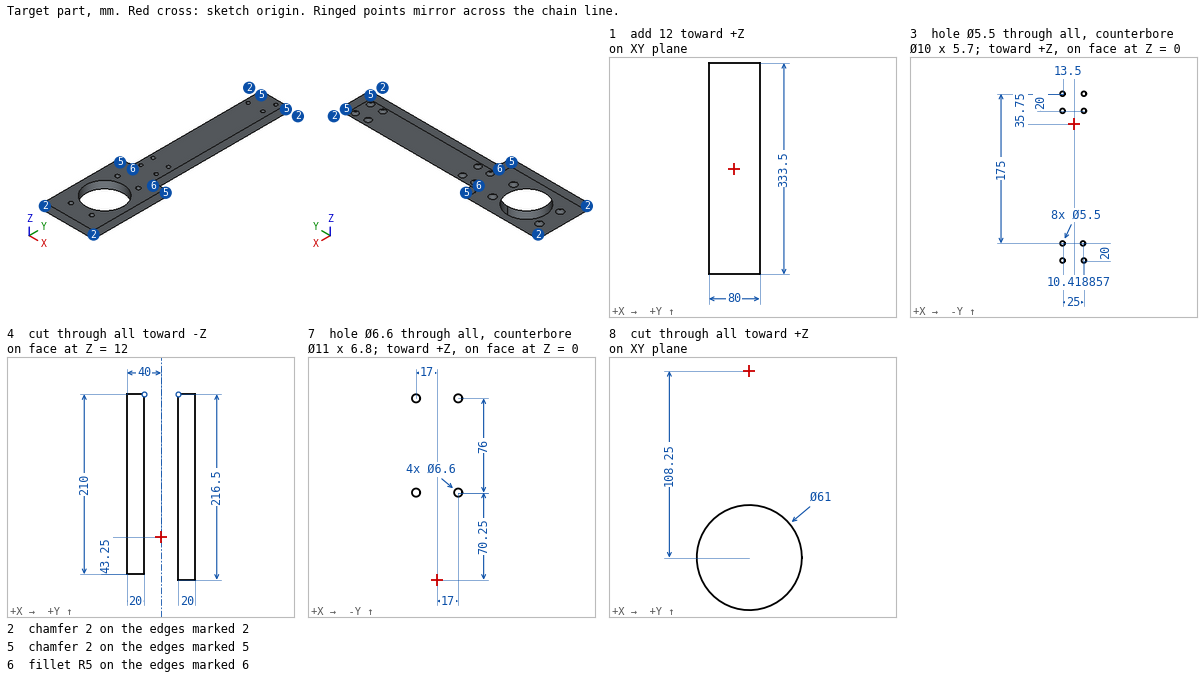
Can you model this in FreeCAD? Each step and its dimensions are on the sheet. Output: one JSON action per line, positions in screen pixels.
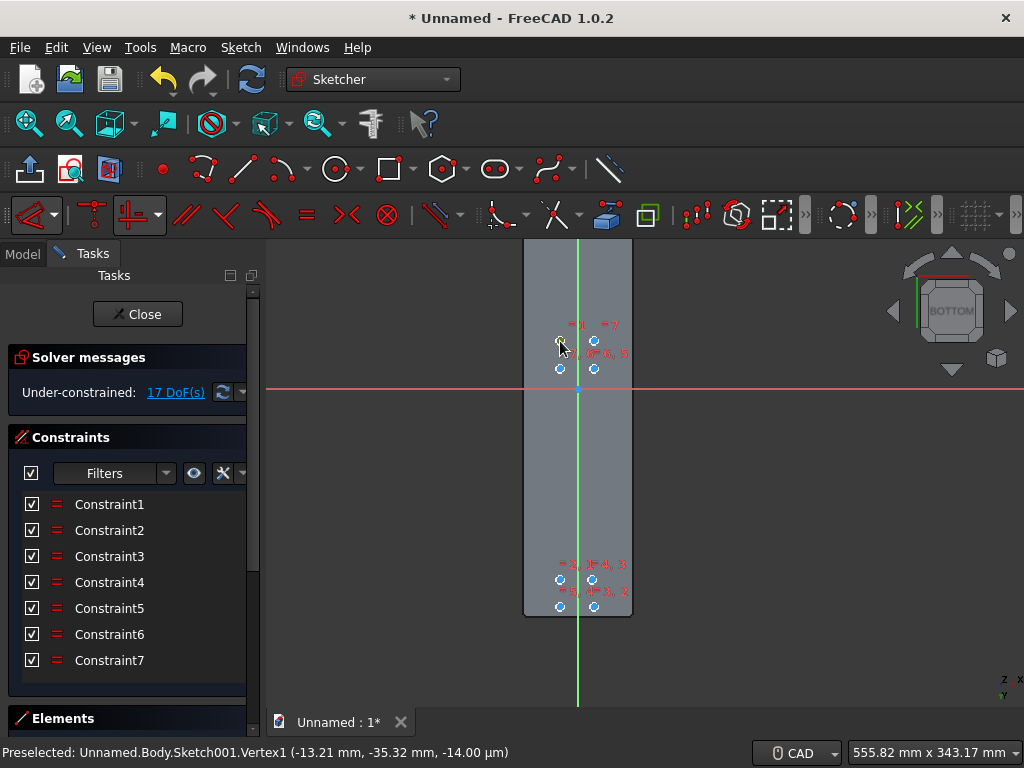
{"action": "left_click", "coordinate": [560, 580]}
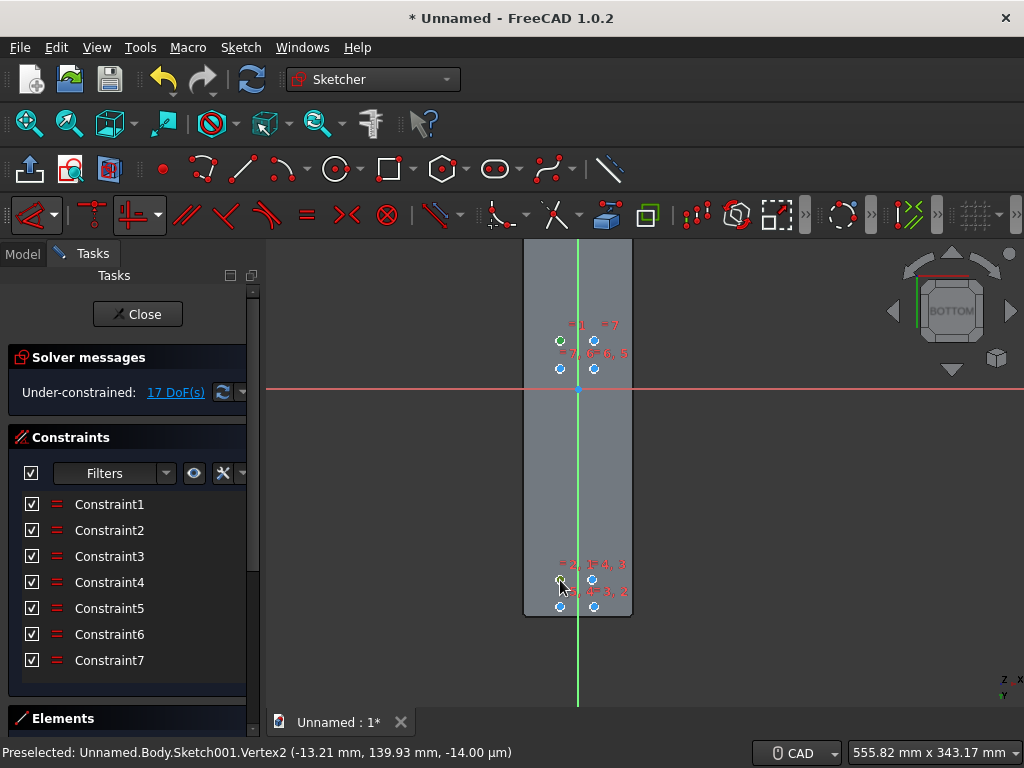
{"action": "key", "text": "v"}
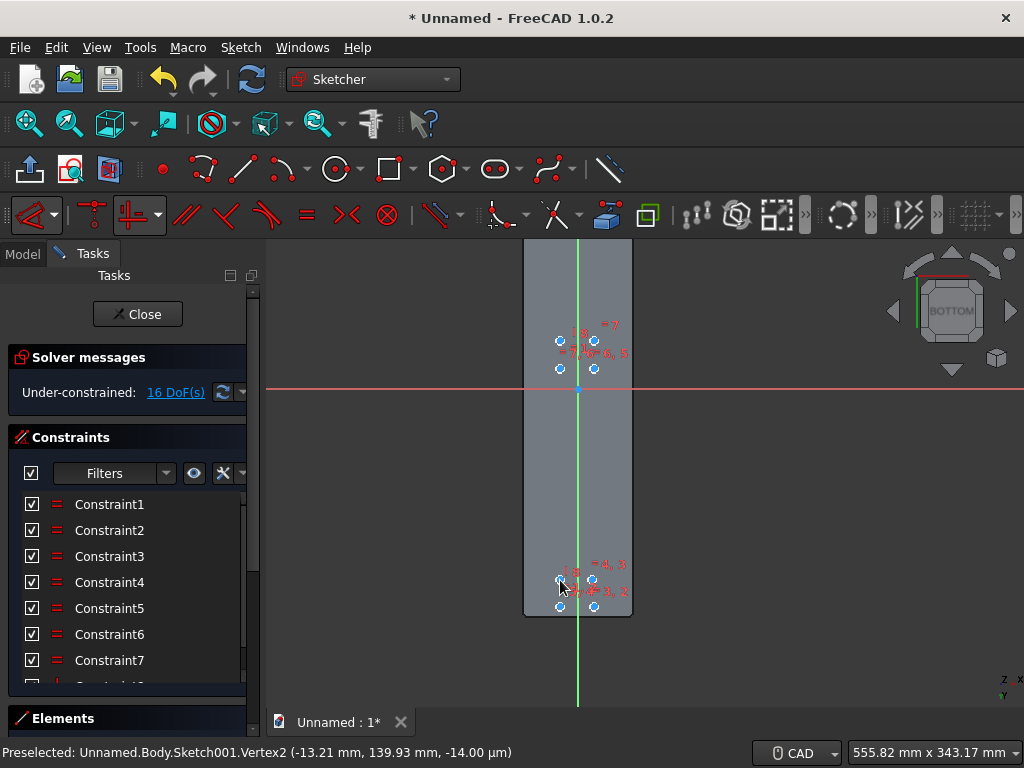
{"action": "left_click", "coordinate": [560, 580]}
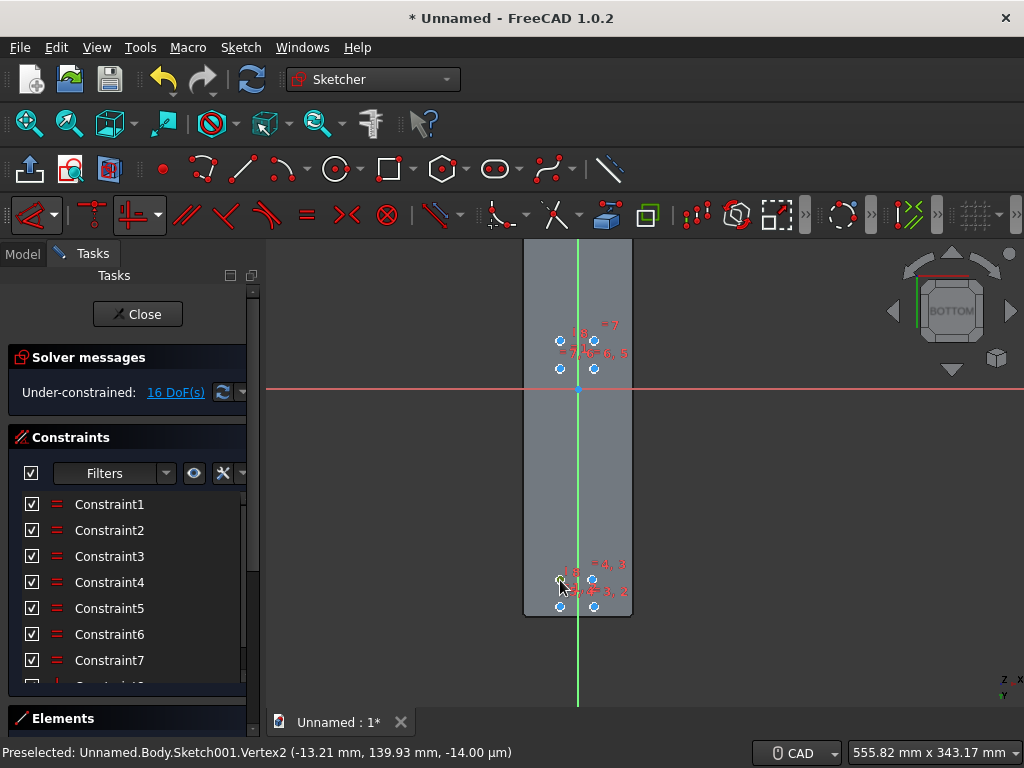
{"action": "scroll", "coordinate": [592, 580], "scroll_direction": "up", "scroll_amount": 4}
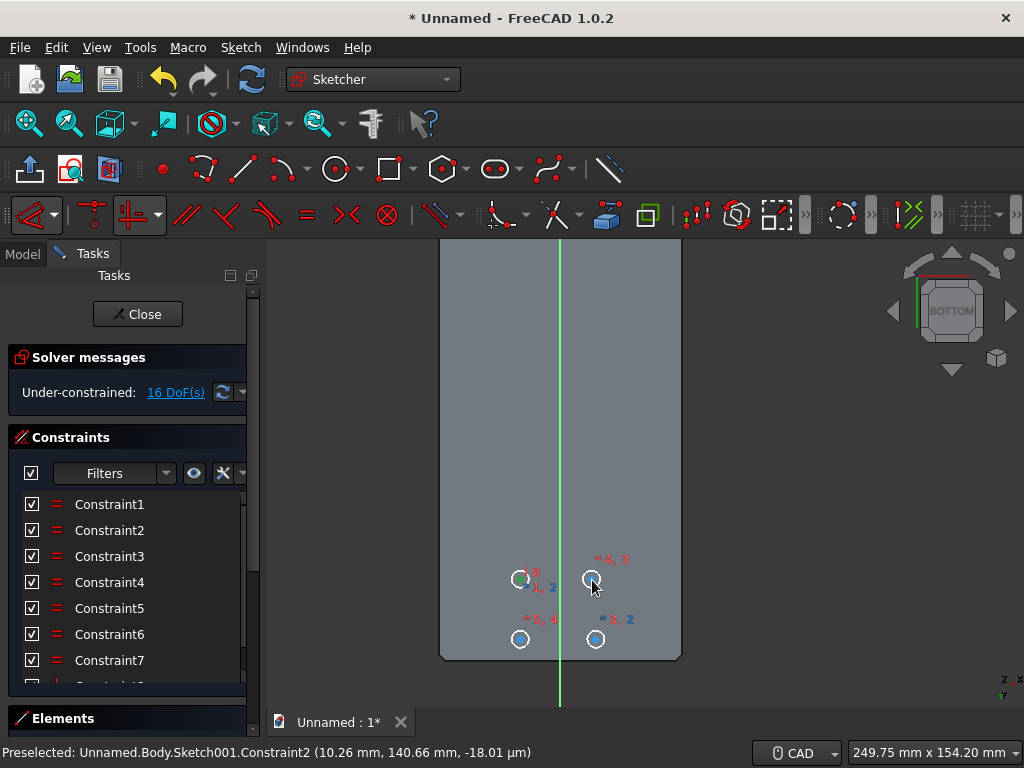
{"action": "left_click", "coordinate": [591, 579]}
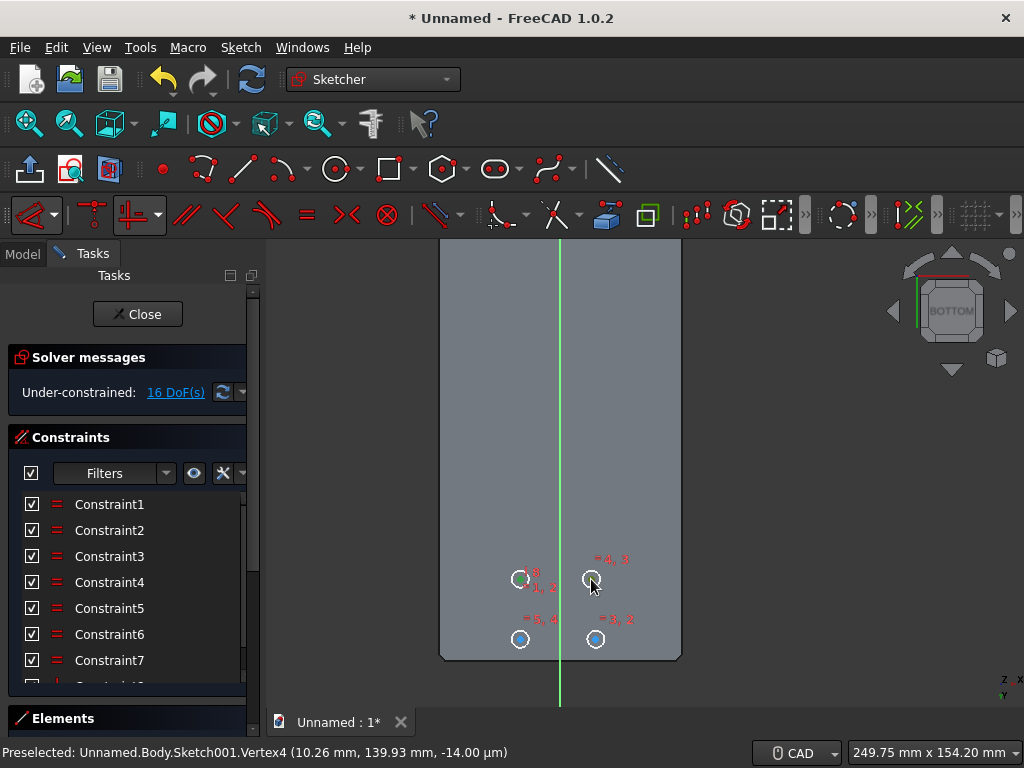
{"action": "left_click", "coordinate": [160, 216]}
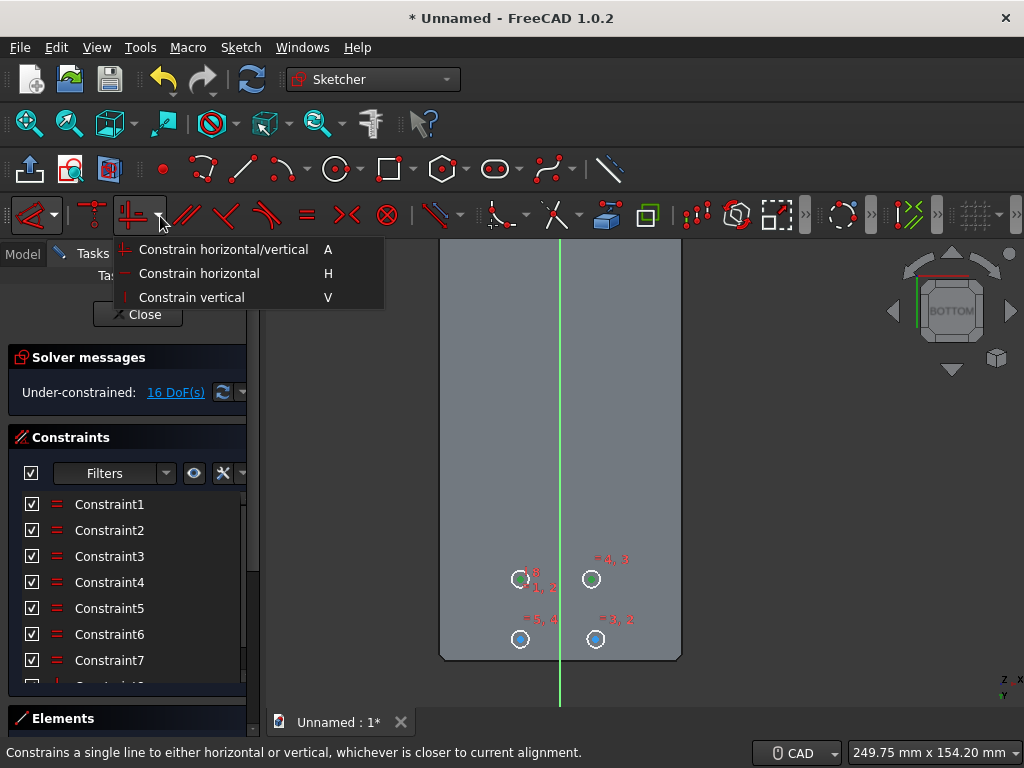
{"action": "left_click", "coordinate": [249, 273]}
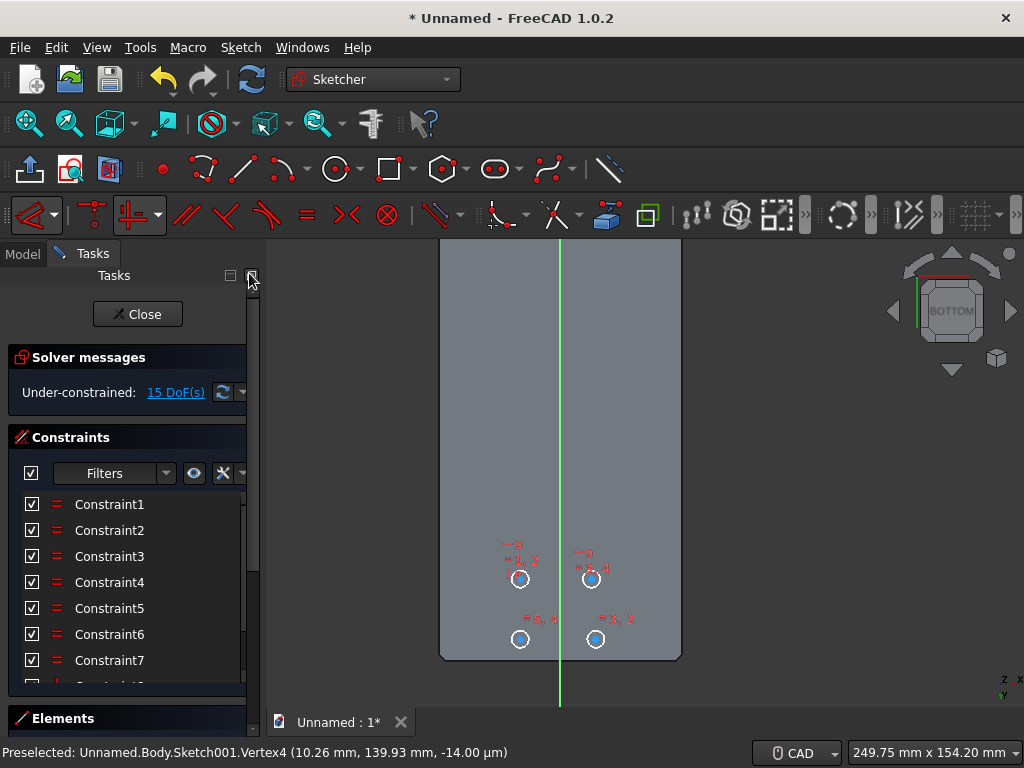
{"action": "left_click", "coordinate": [520, 579]}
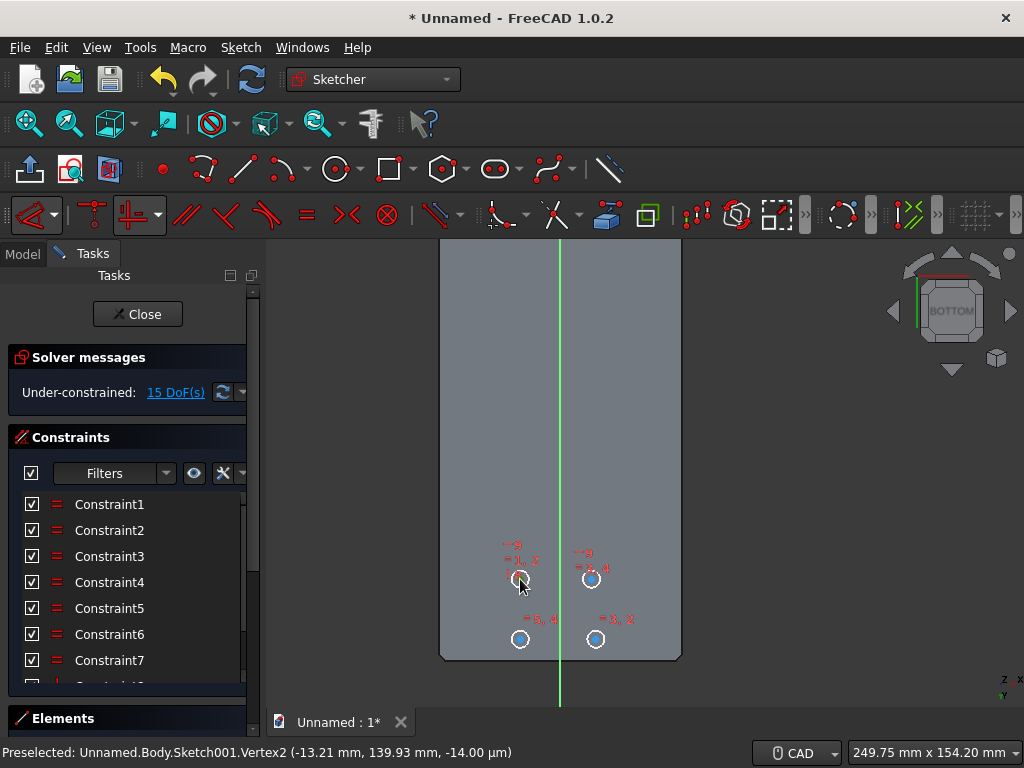
{"action": "left_click", "coordinate": [520, 639]}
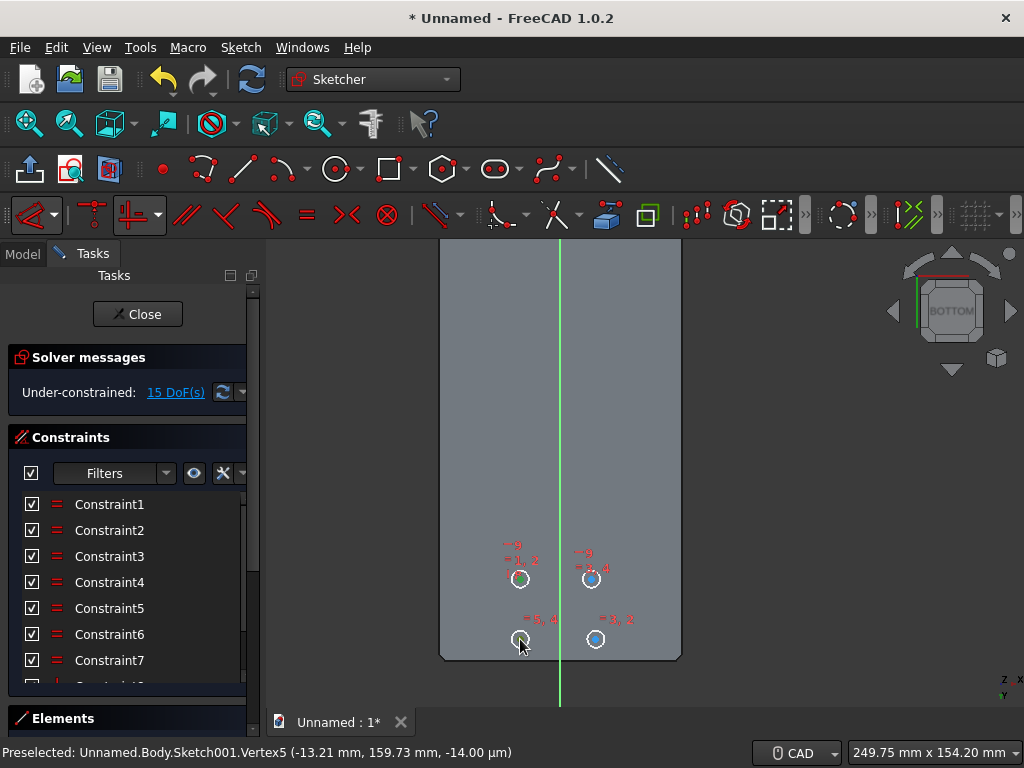
{"action": "left_click", "coordinate": [160, 216]}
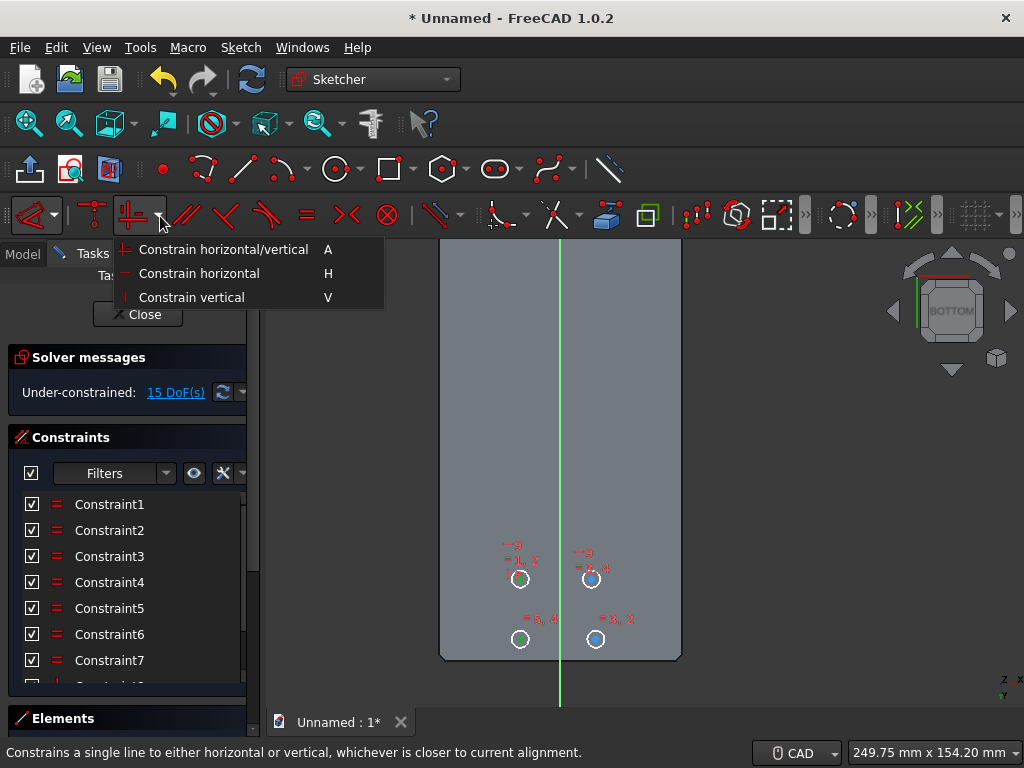
{"action": "left_click", "coordinate": [249, 297]}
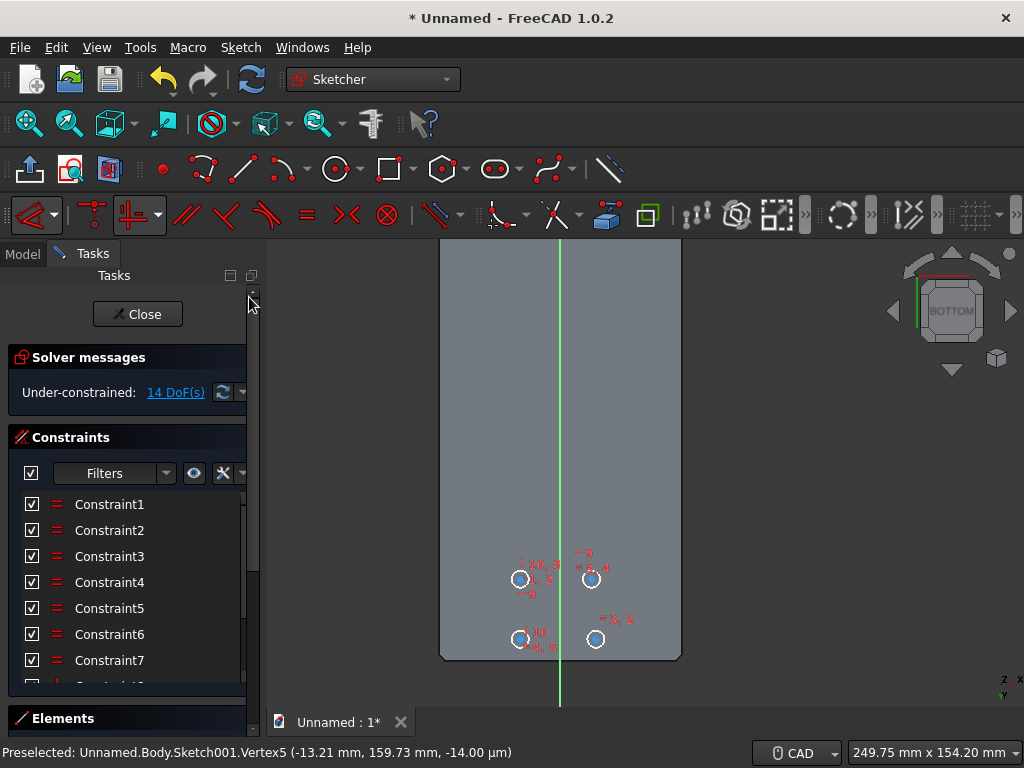
{"action": "left_click", "coordinate": [596, 639]}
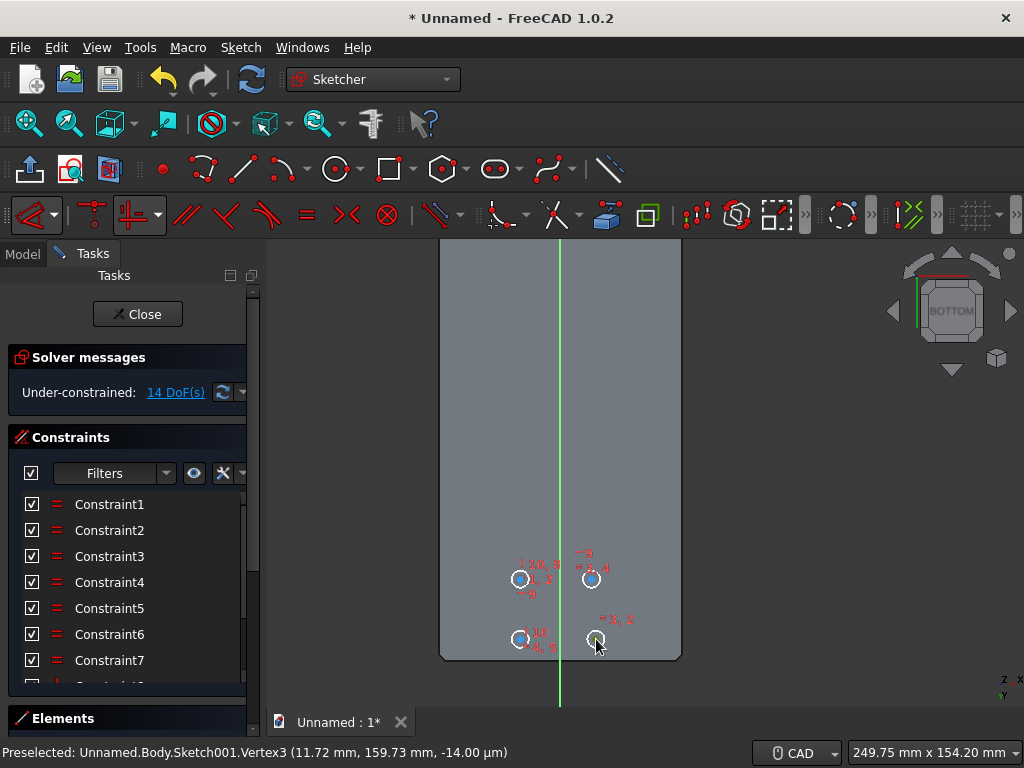
{"action": "left_click", "coordinate": [520, 639]}